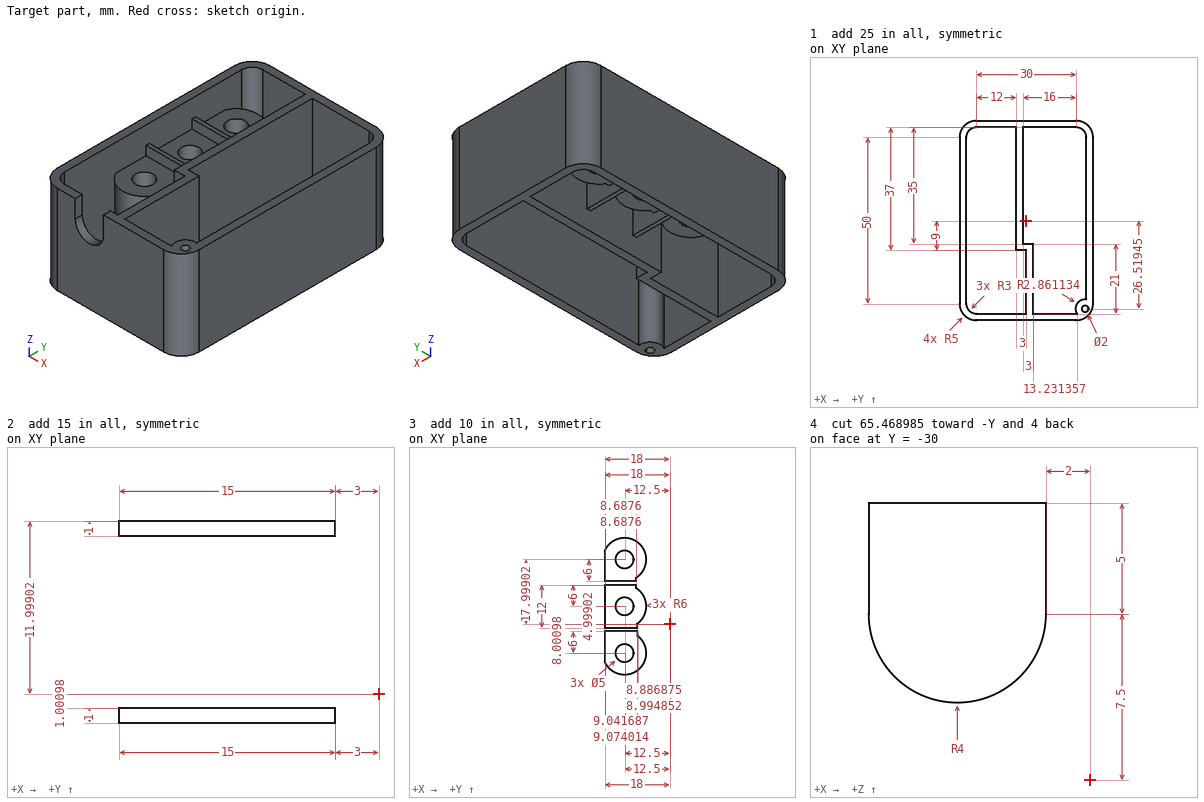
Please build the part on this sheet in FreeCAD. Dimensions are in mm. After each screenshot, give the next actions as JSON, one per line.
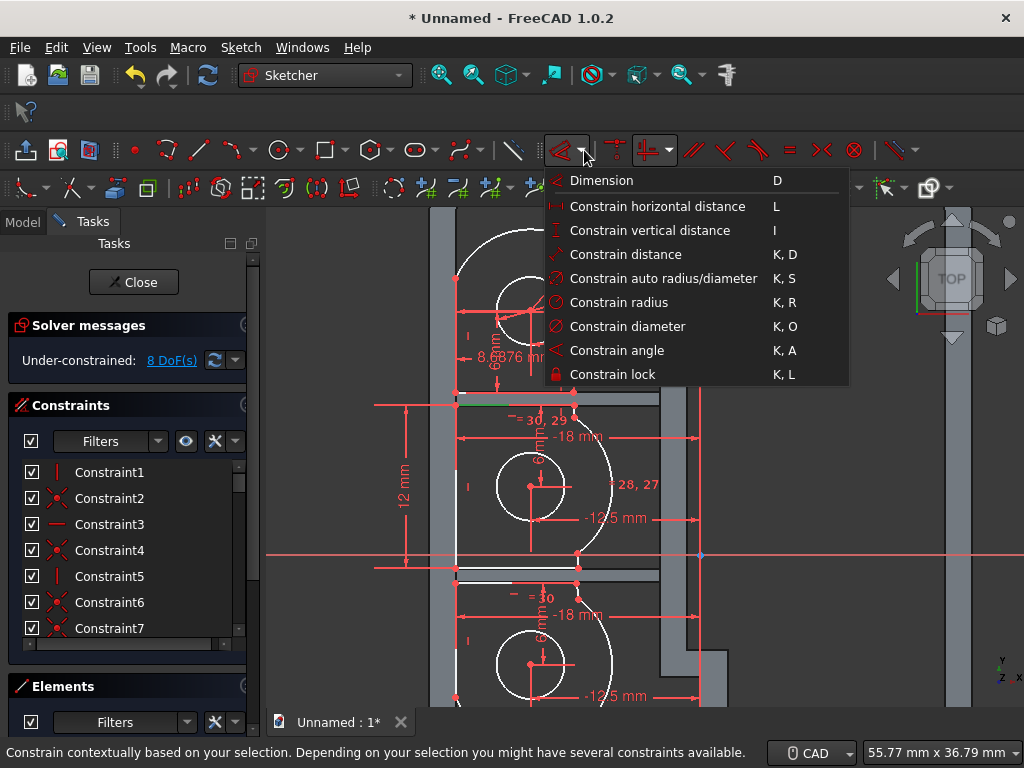
{"action": "left_click", "coordinate": [697, 206]}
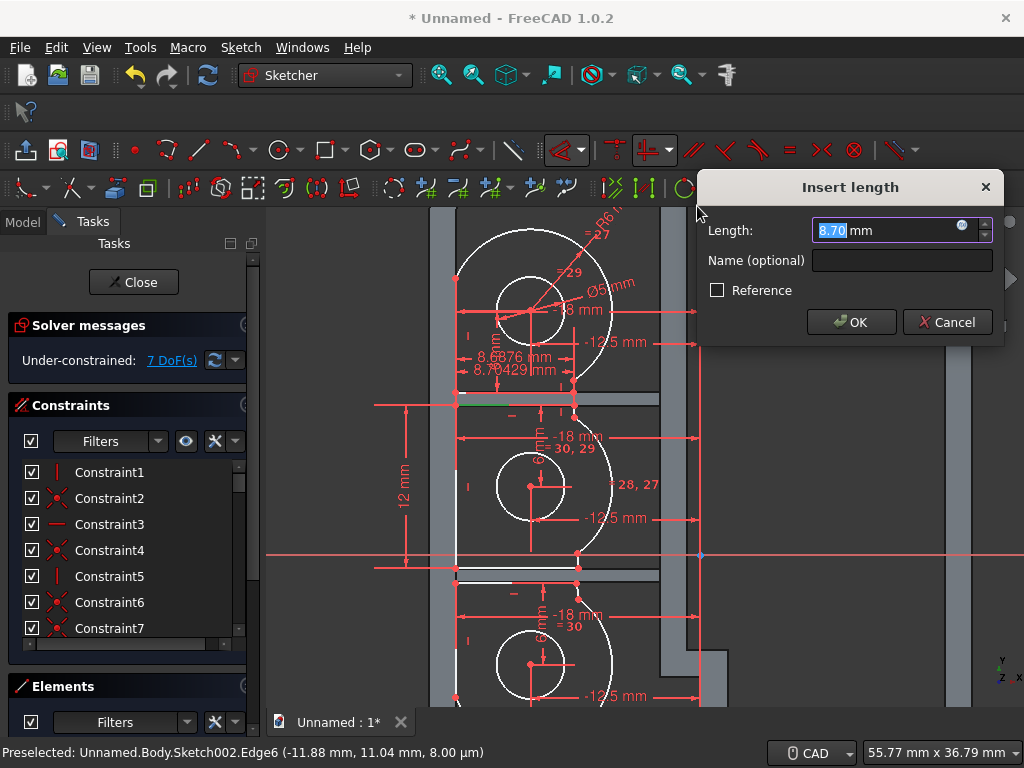
{"action": "type", "text": "8.6876"}
{"action": "key", "text": "Return"}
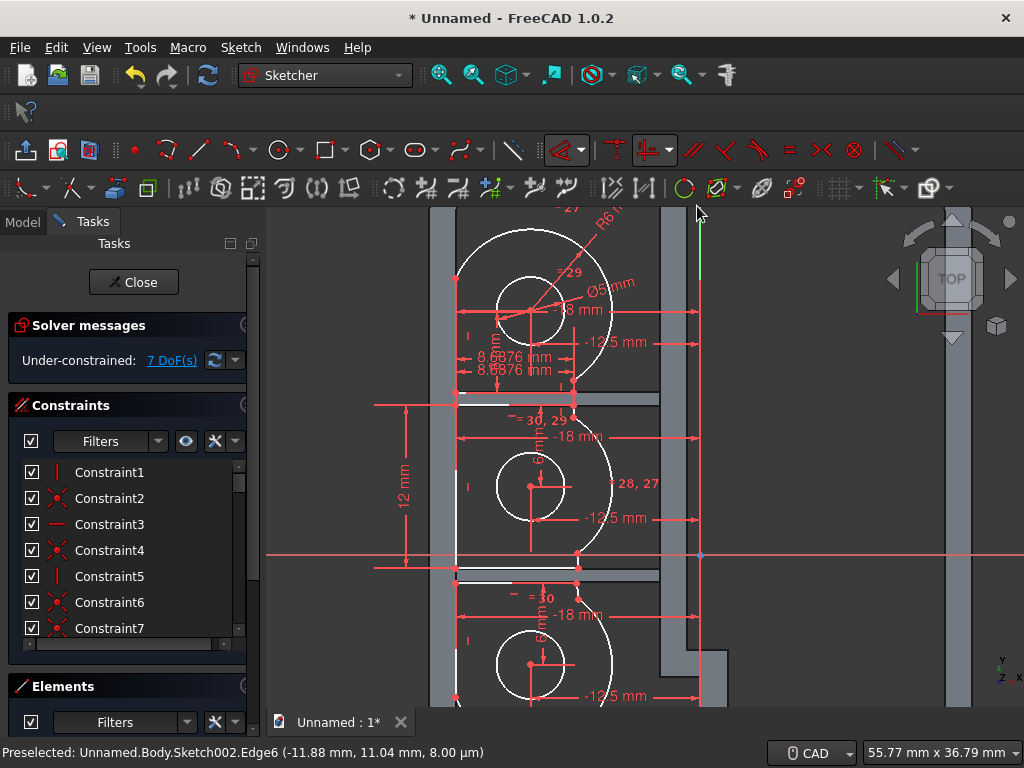
{"action": "left_click", "coordinate": [531, 487]}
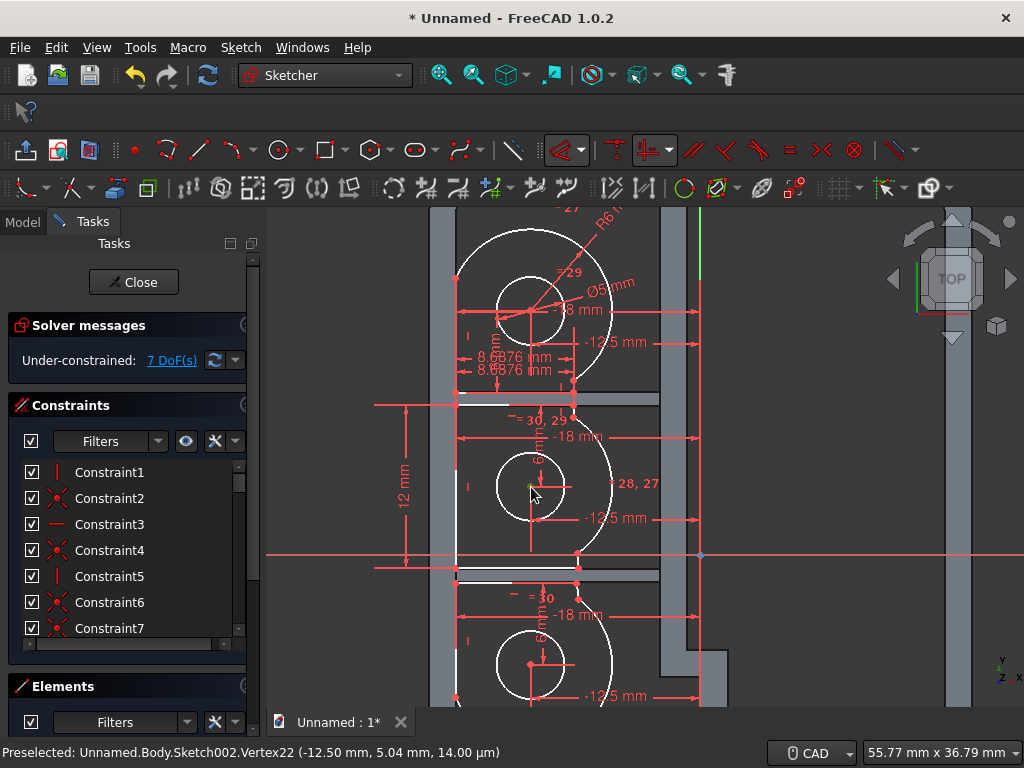
{"action": "left_click", "coordinate": [584, 150]}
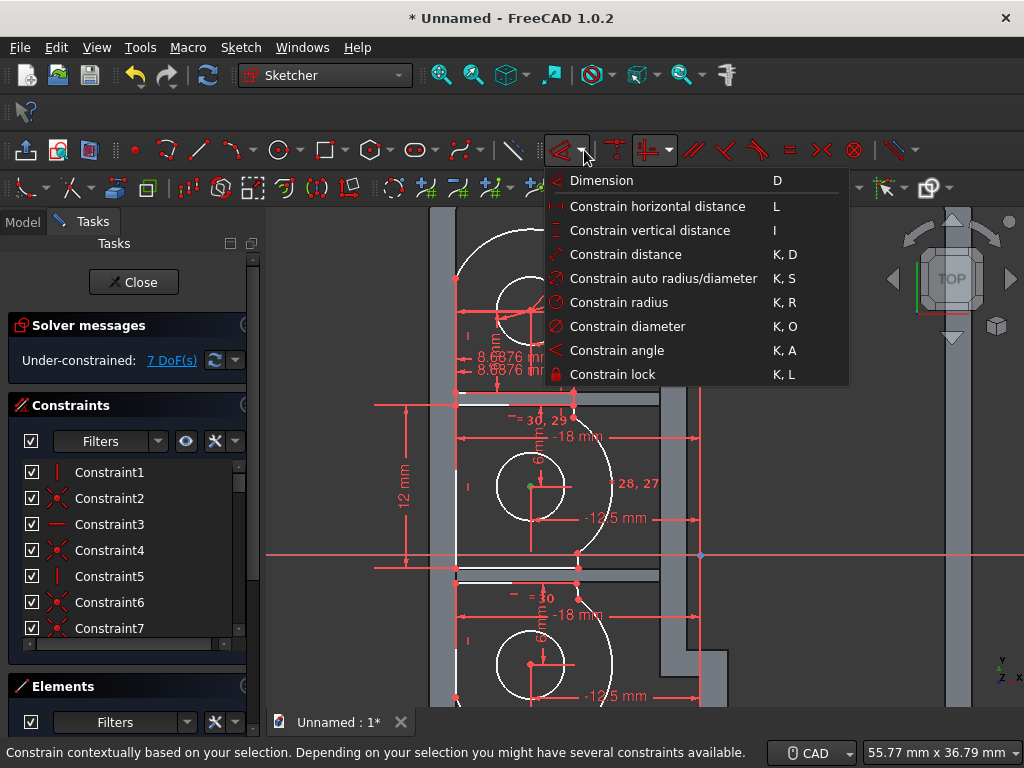
{"action": "left_click", "coordinate": [697, 230]}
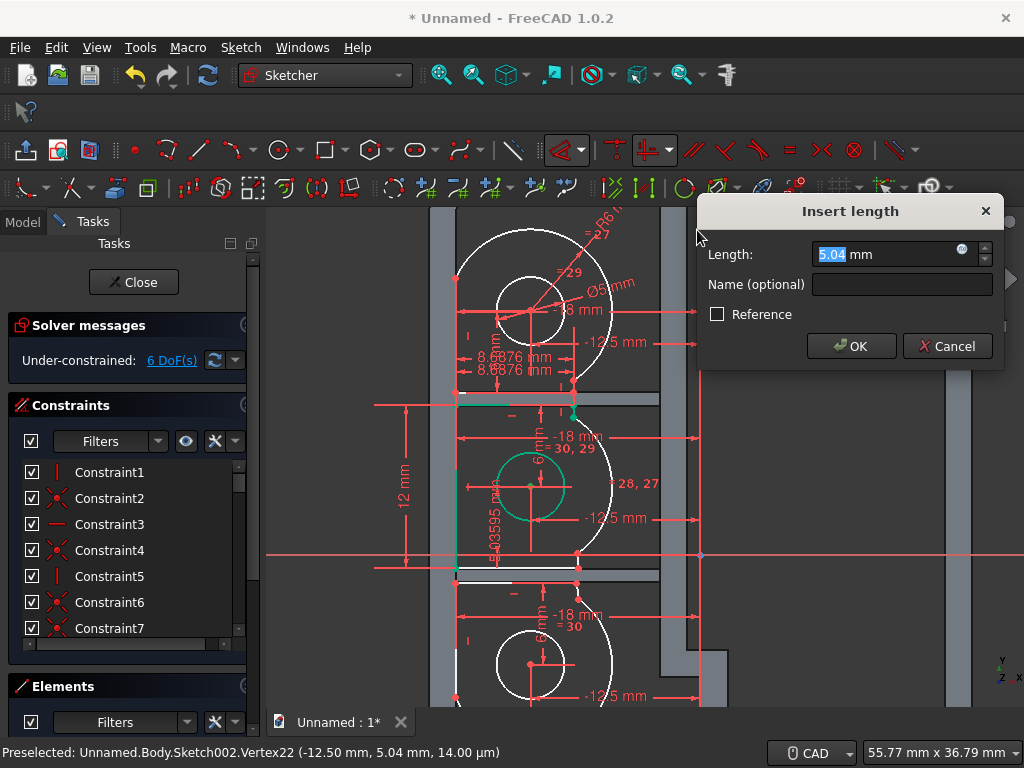
{"action": "type", "text": "4.99902"}
{"action": "key", "text": "Return"}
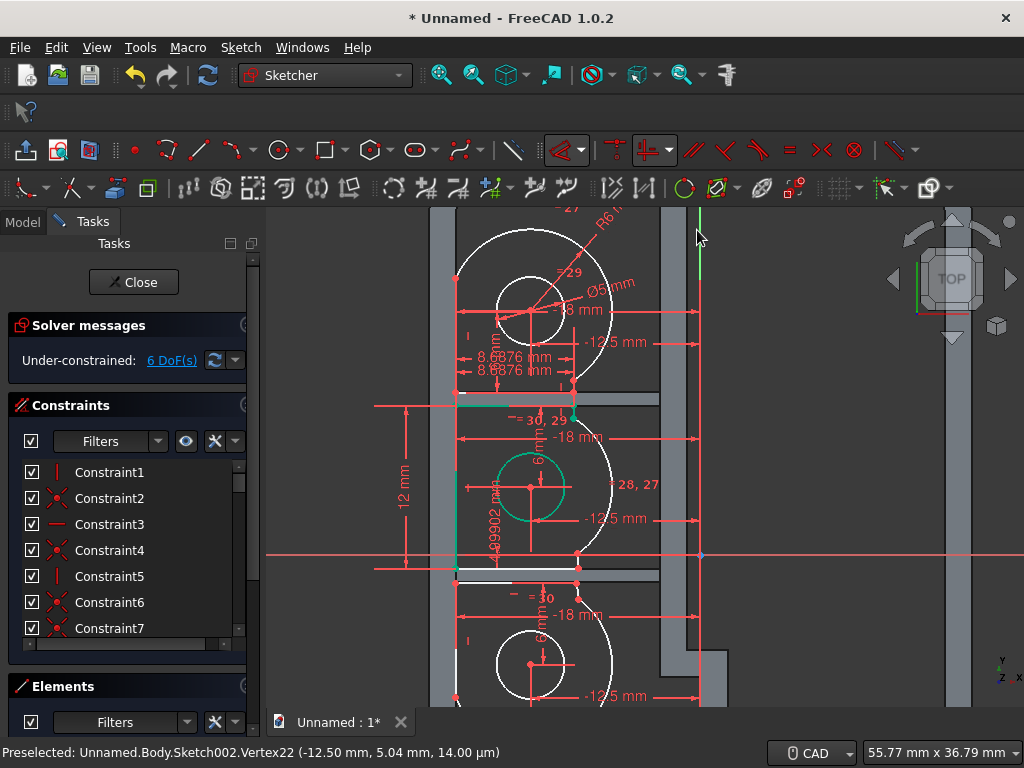
{"action": "left_click", "coordinate": [531, 665]}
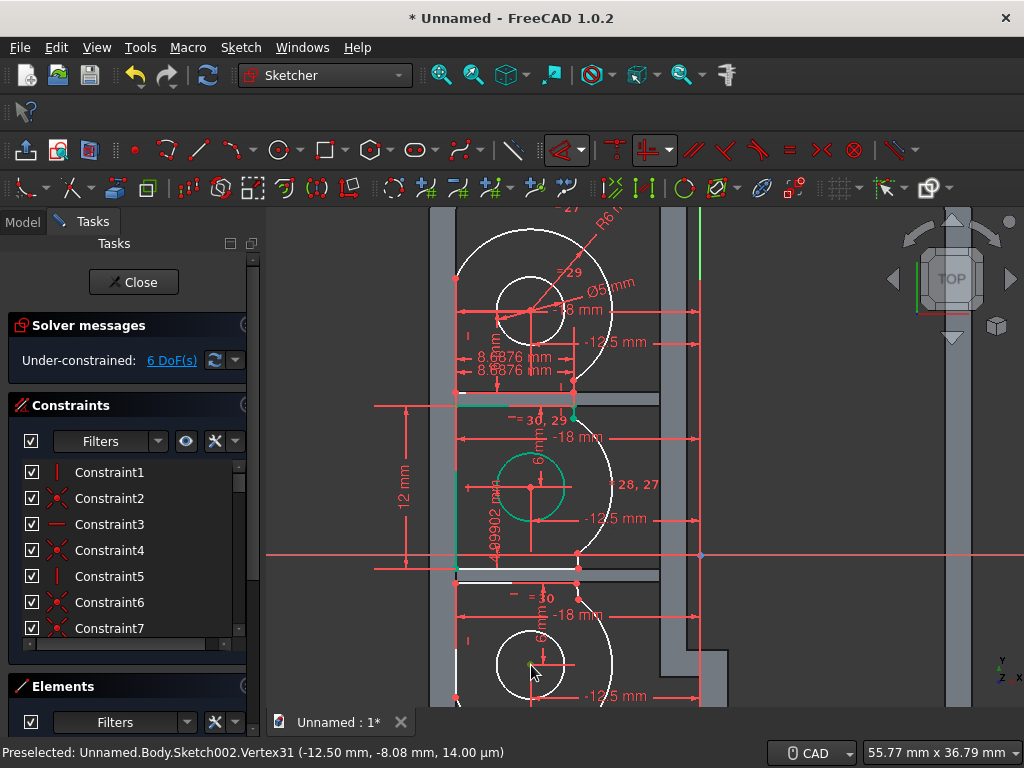
{"action": "key", "text": "i"}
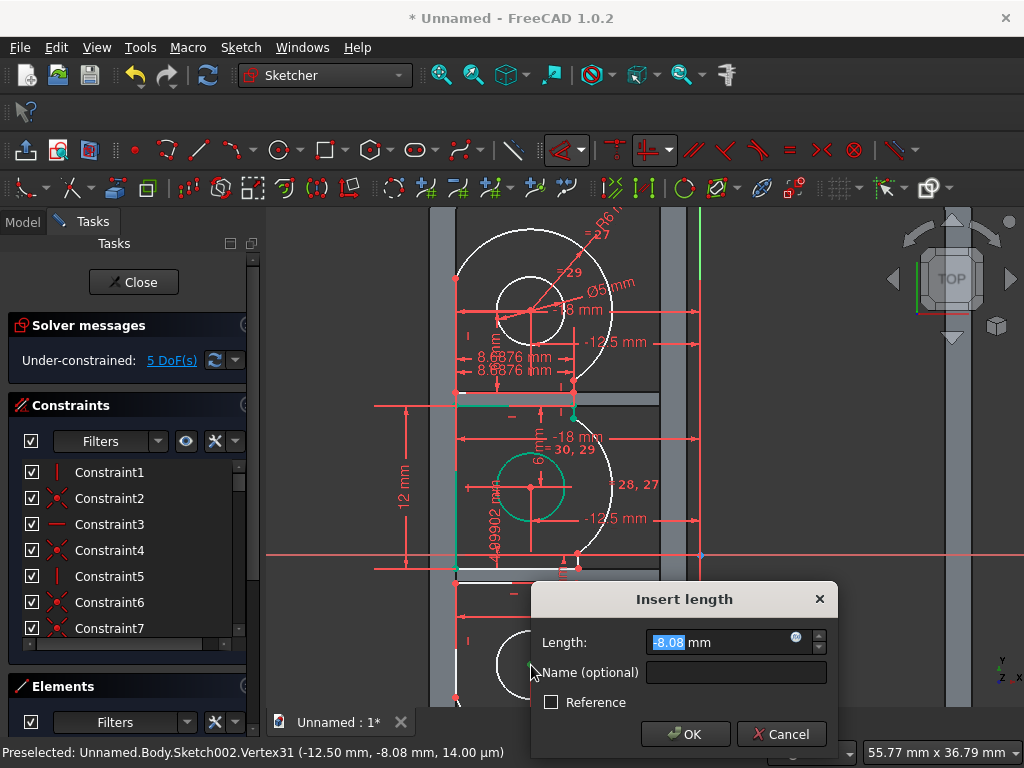
{"action": "type", "text": "-8.00098"}
{"action": "key", "text": "Return"}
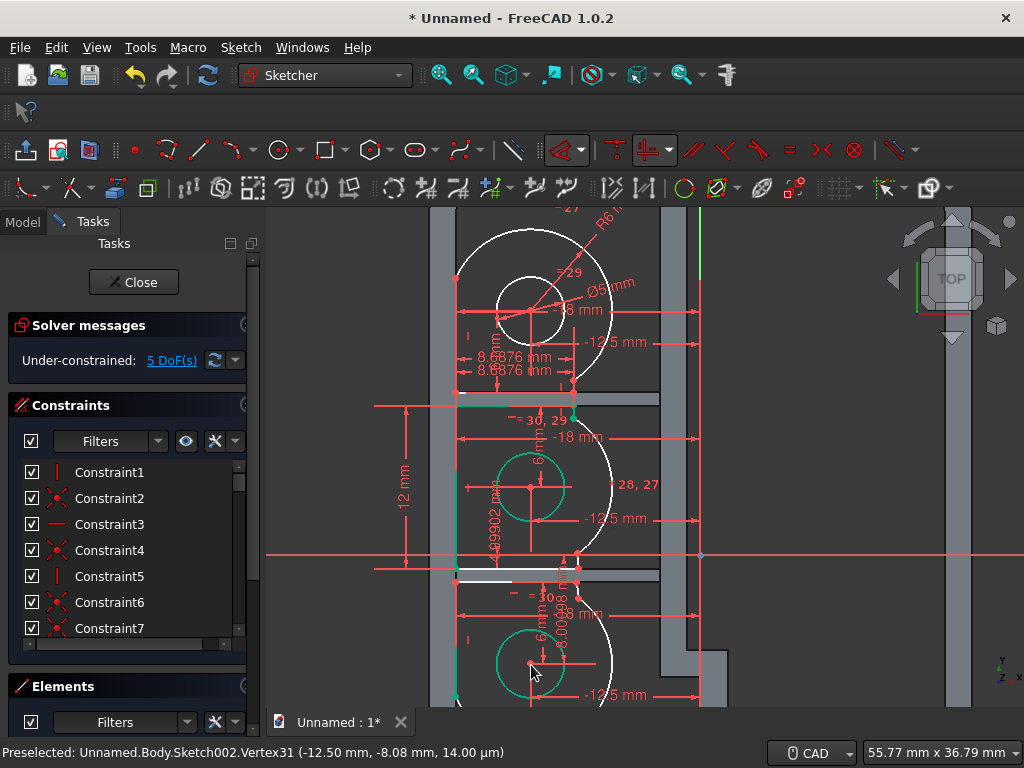
{"action": "left_click", "coordinate": [493, 569]}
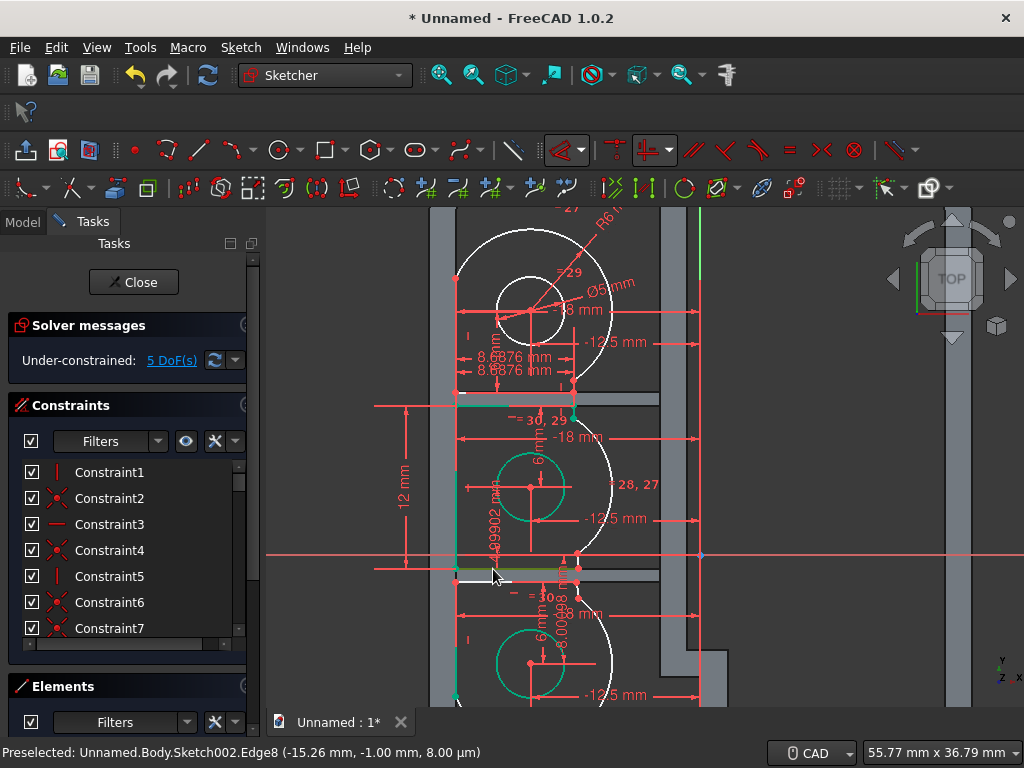
{"action": "left_click", "coordinate": [584, 150]}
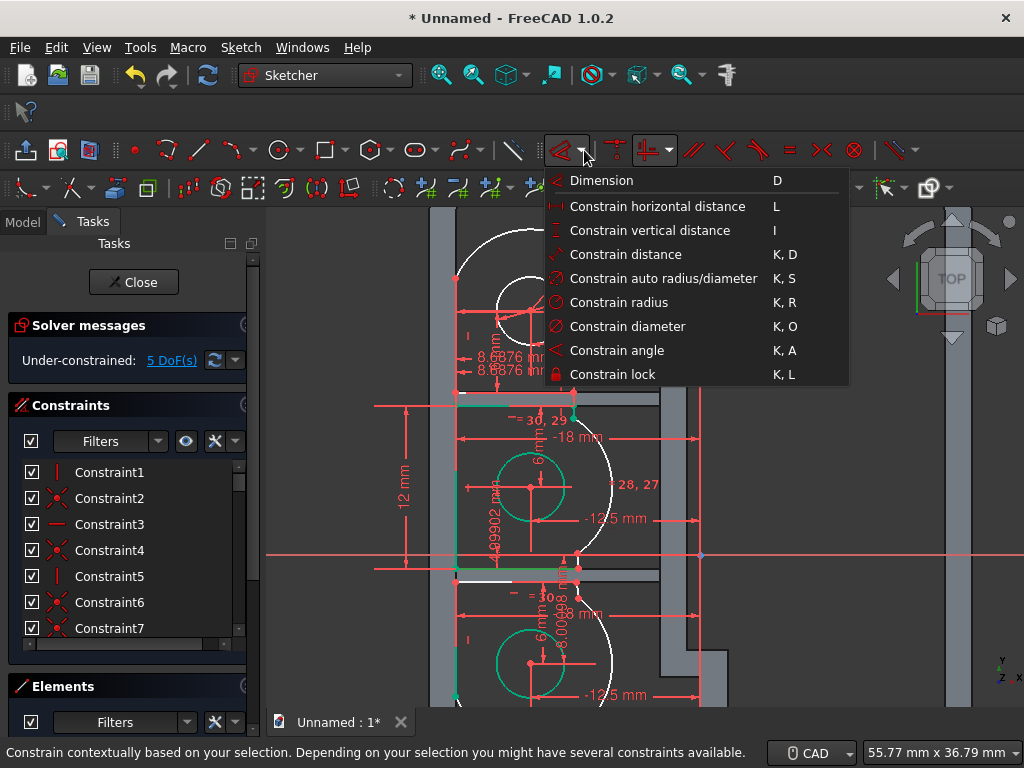
{"action": "left_click", "coordinate": [697, 206]}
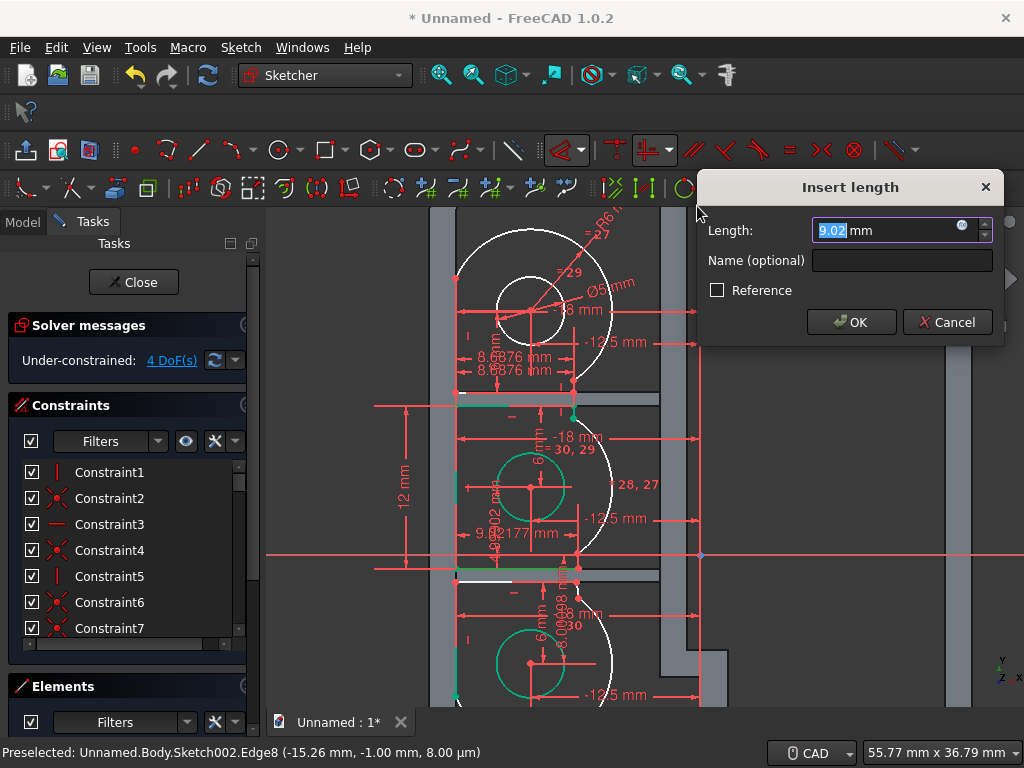
{"action": "type", "text": "9.041687"}
{"action": "key", "text": "Return"}